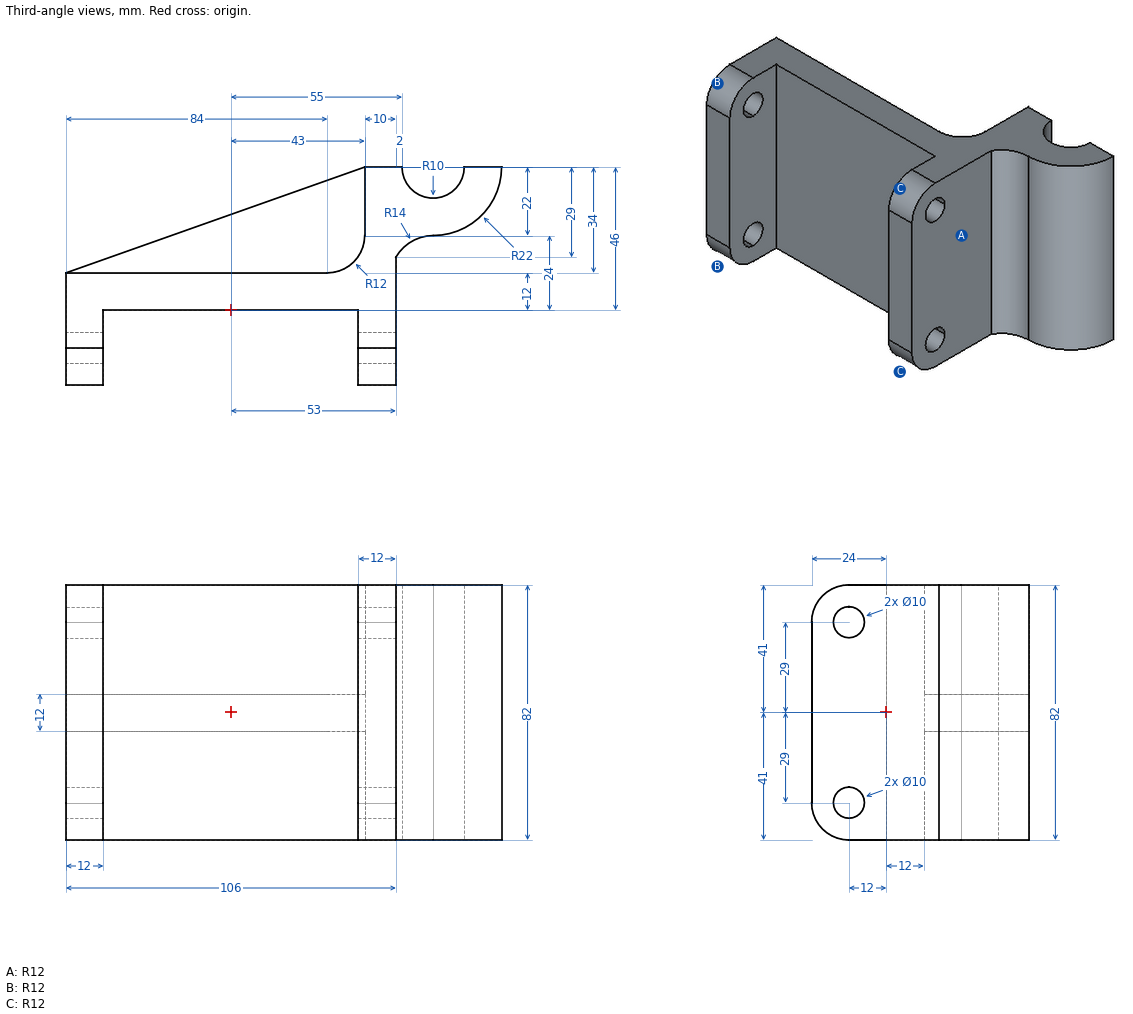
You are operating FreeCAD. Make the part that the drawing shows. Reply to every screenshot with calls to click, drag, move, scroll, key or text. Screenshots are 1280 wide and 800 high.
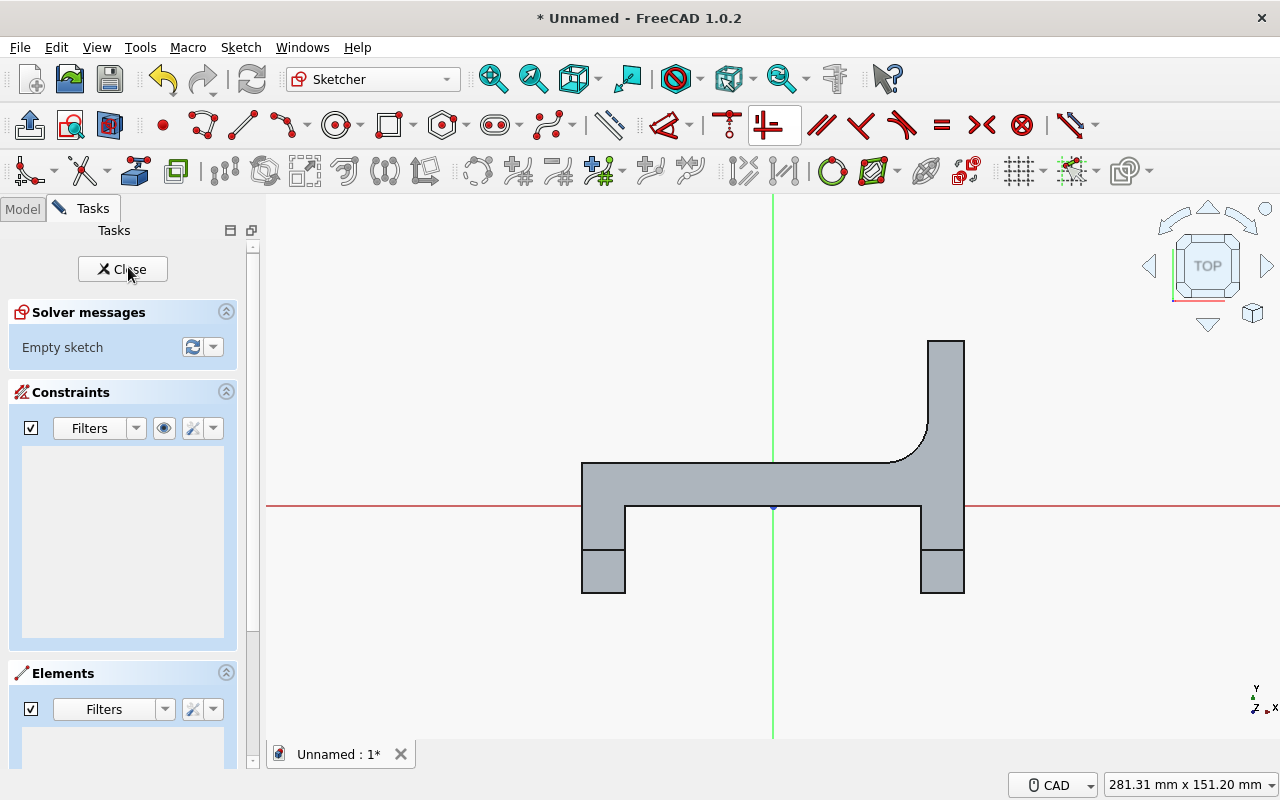
key(q)
key(s)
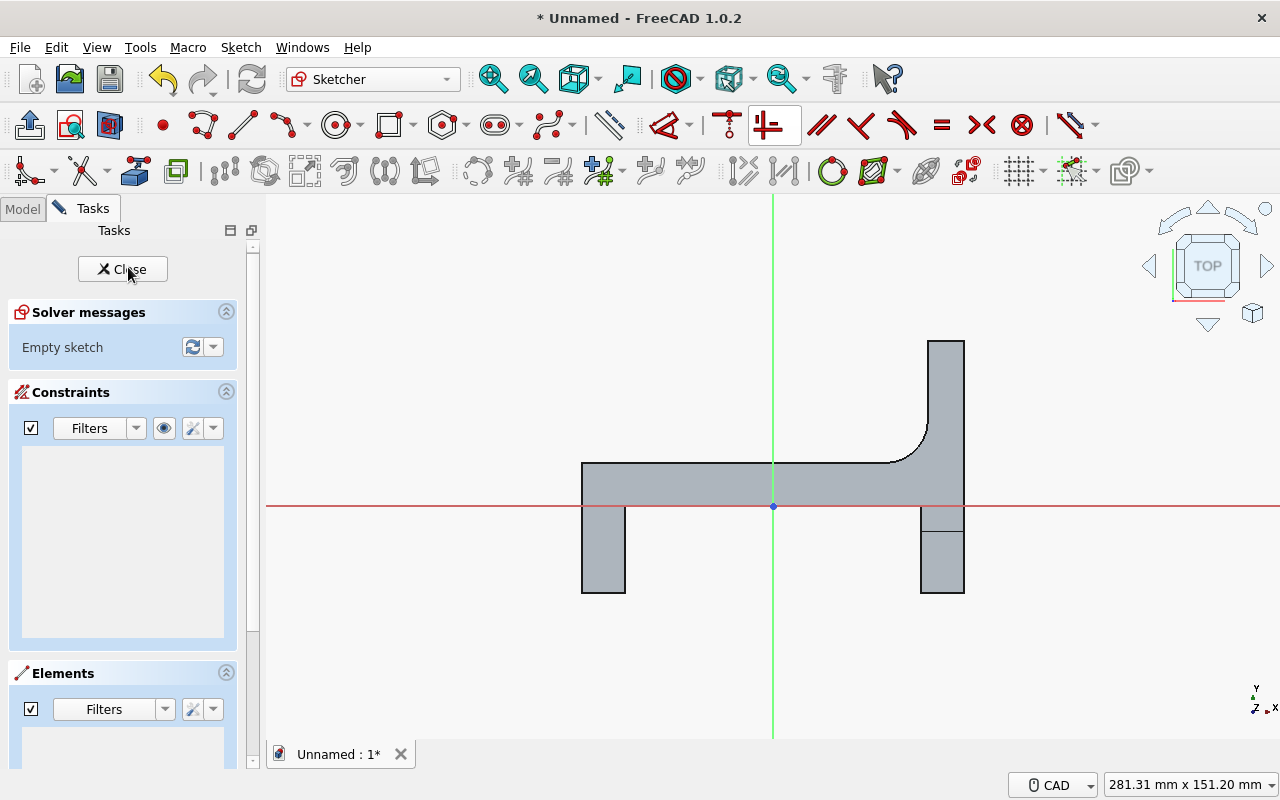
scroll(816, 371, up, 3)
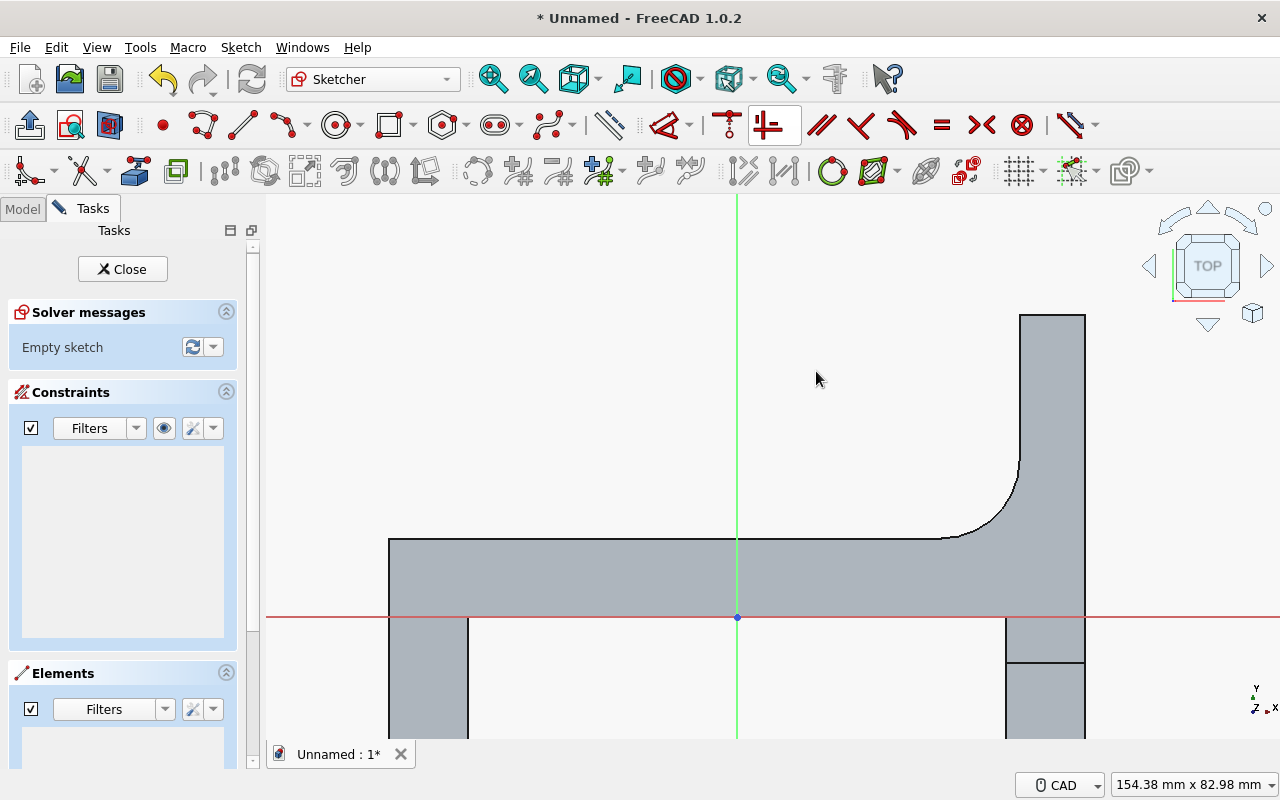
key(g)
key(m)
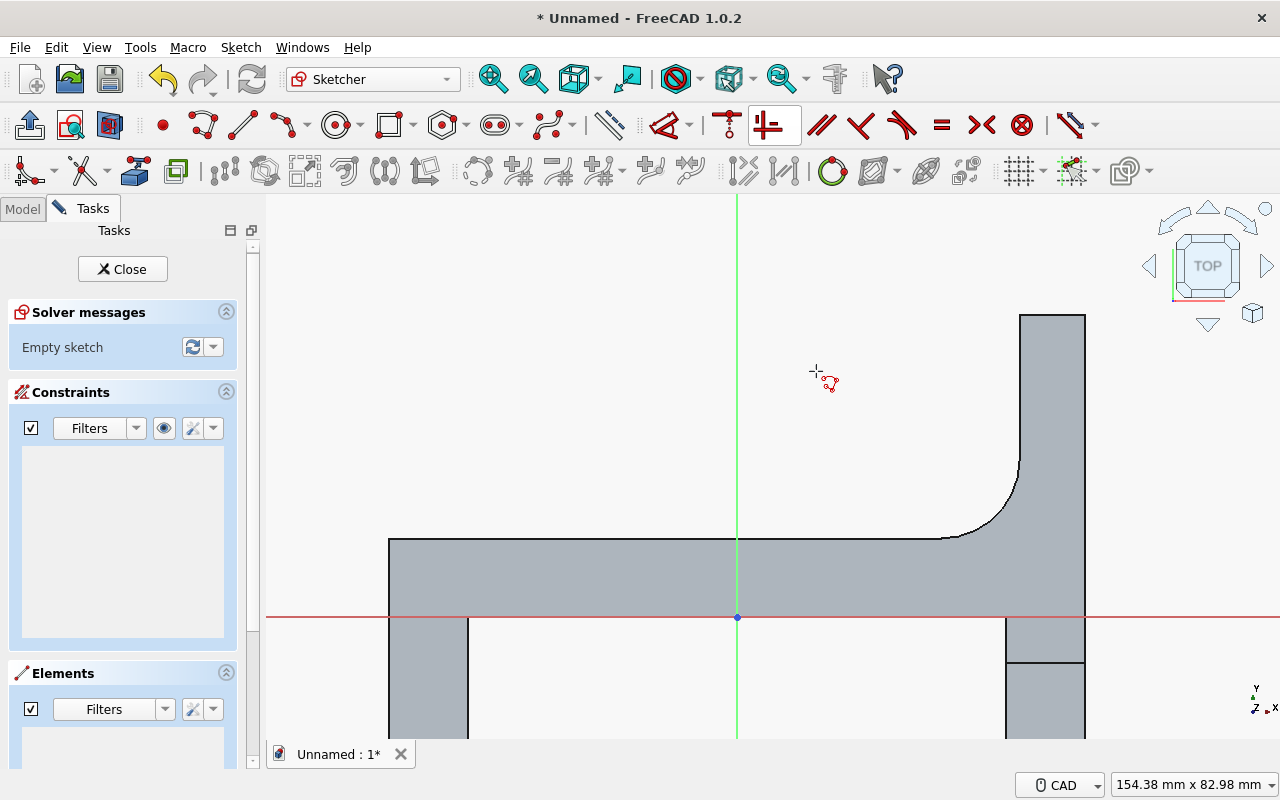
click(1020, 460)
click(1020, 315)
click(389, 539)
click(941, 539)
right_click(941, 539)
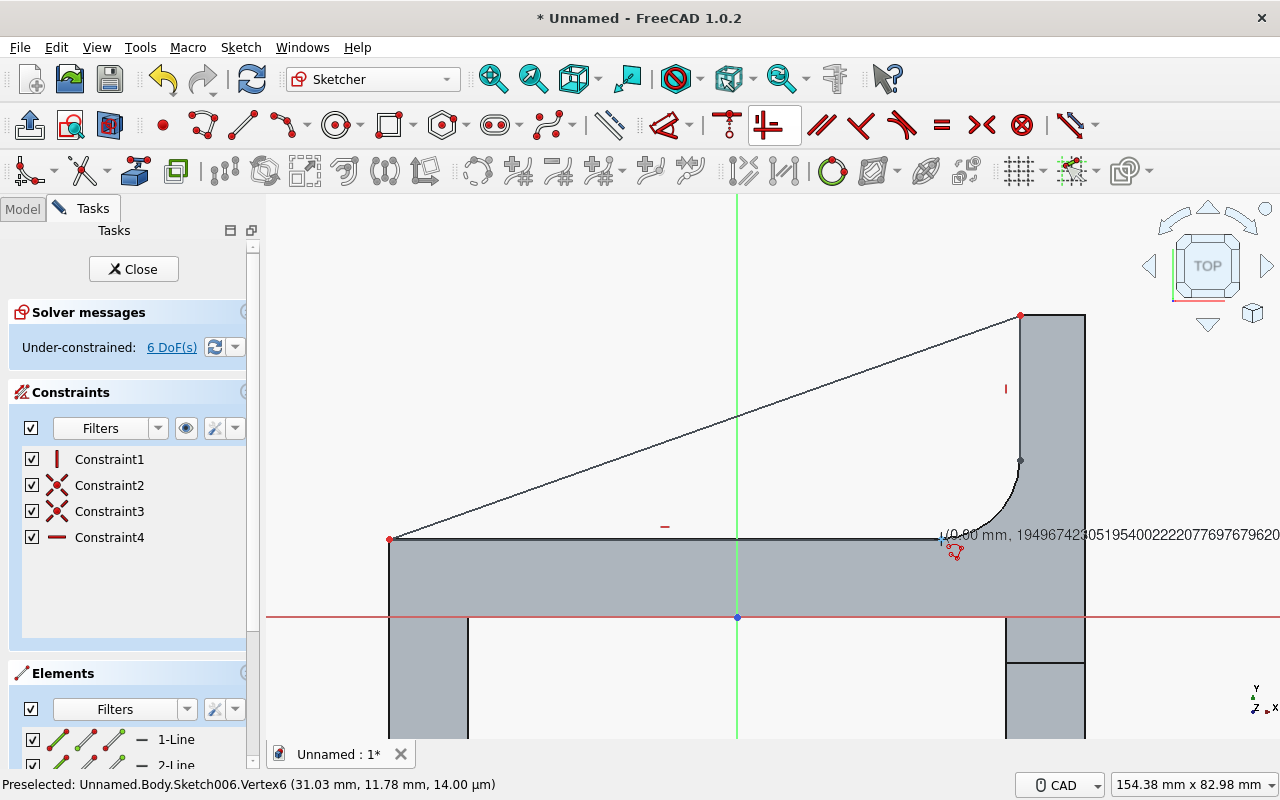
click(284, 126)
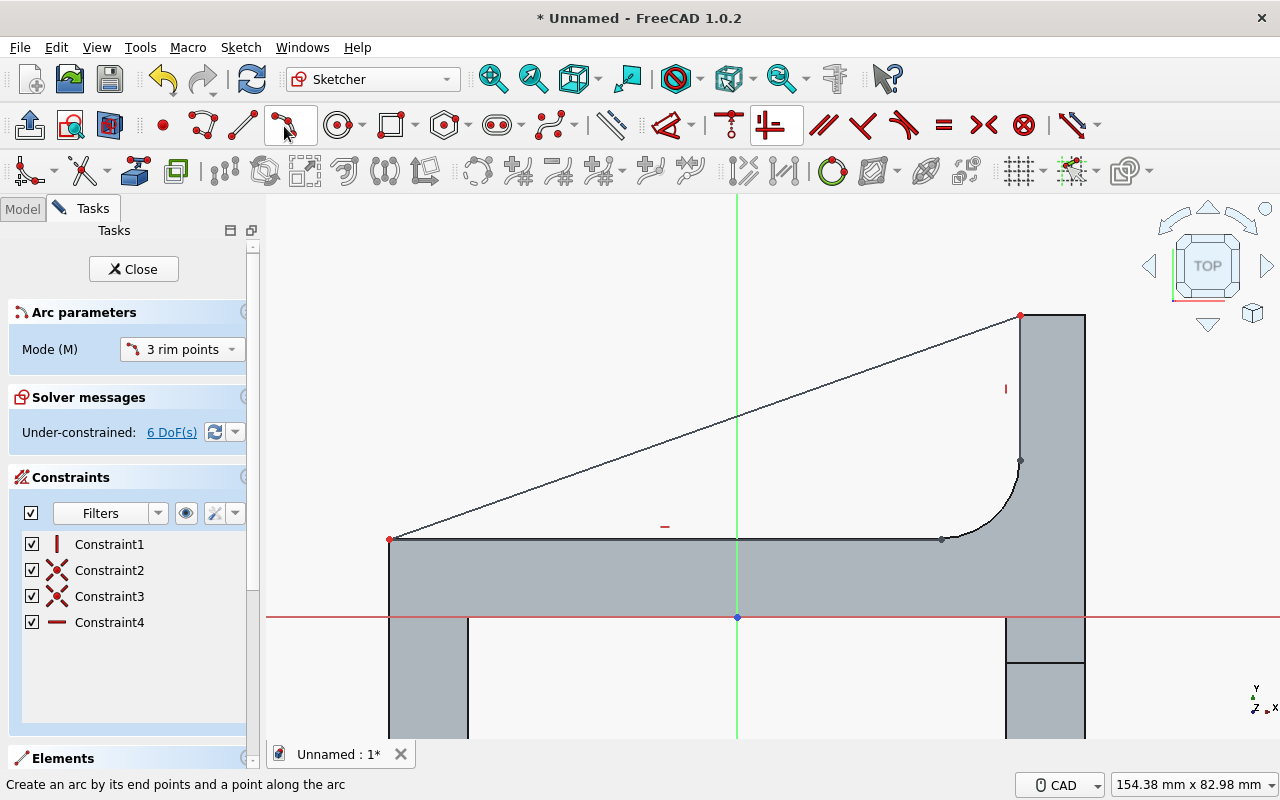
click(941, 540)
click(1020, 461)
click(997, 515)
key(Escape)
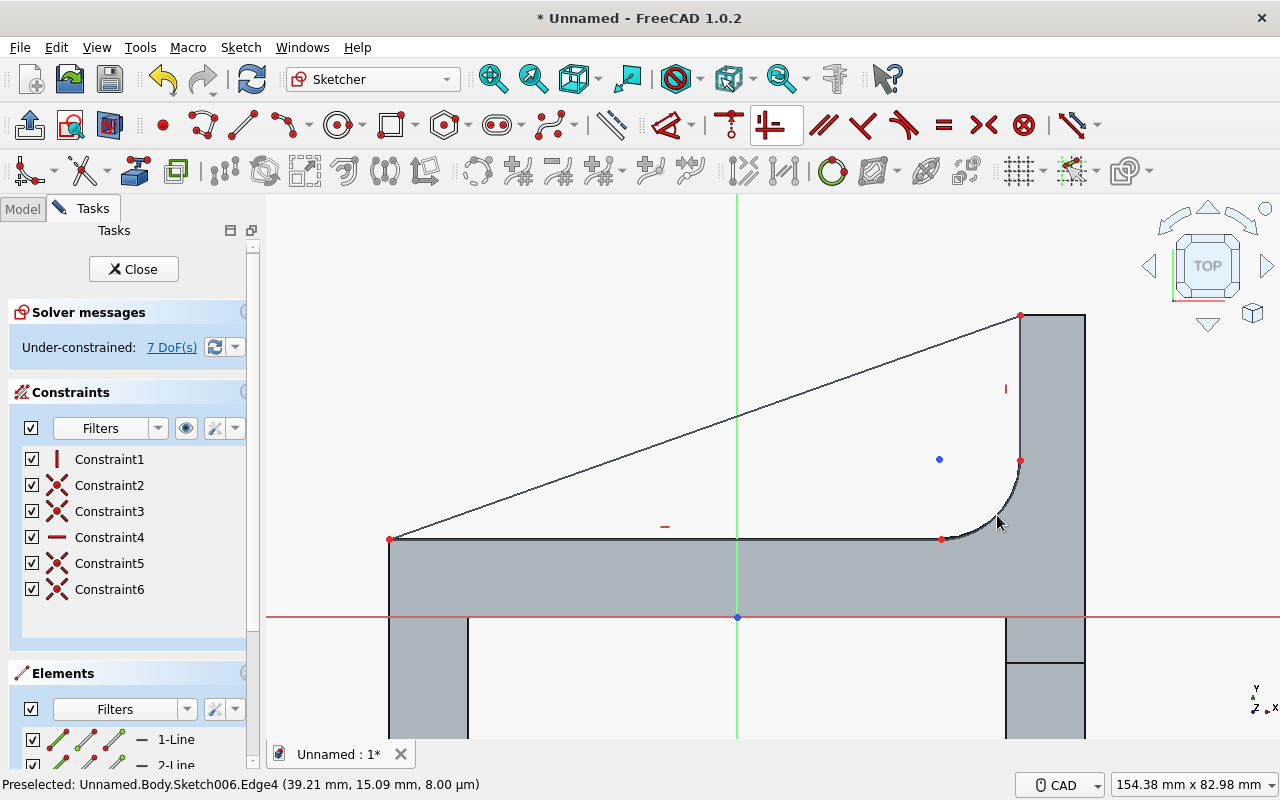
click(1020, 418)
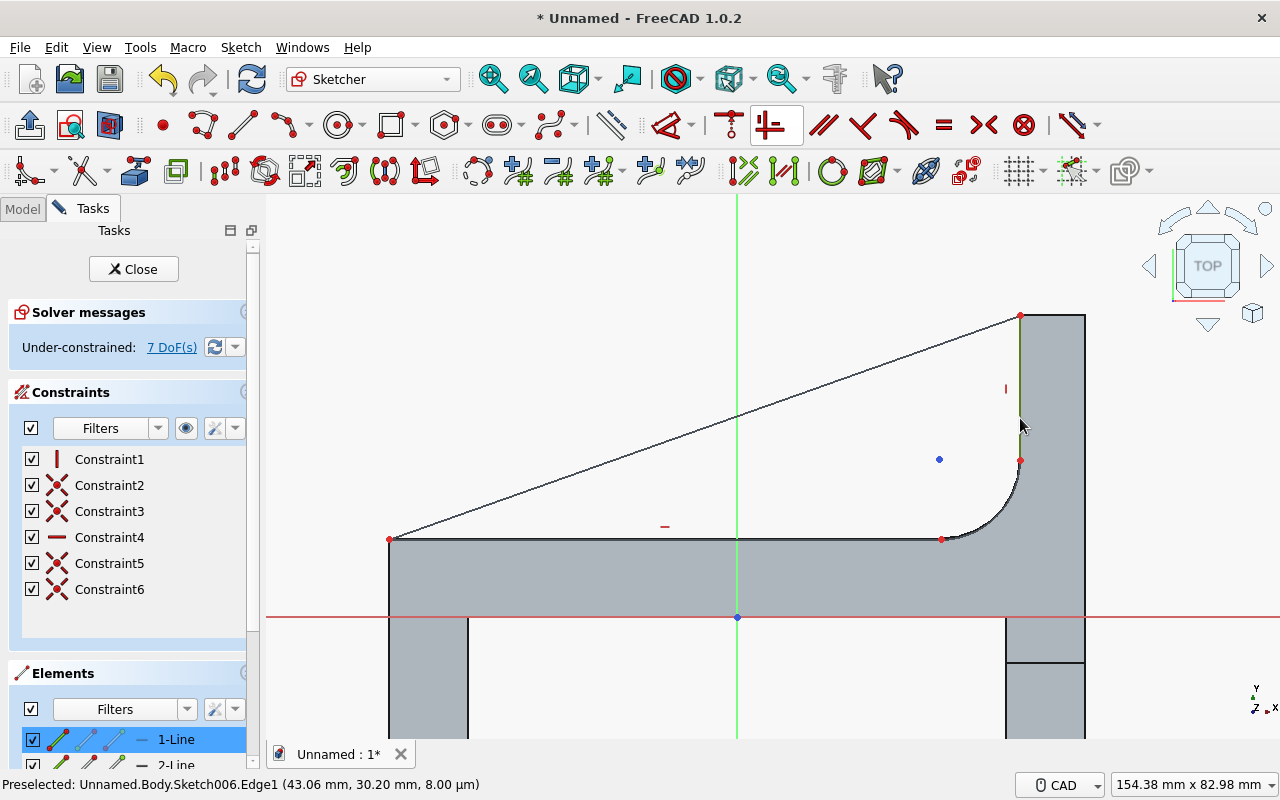
click(977, 531)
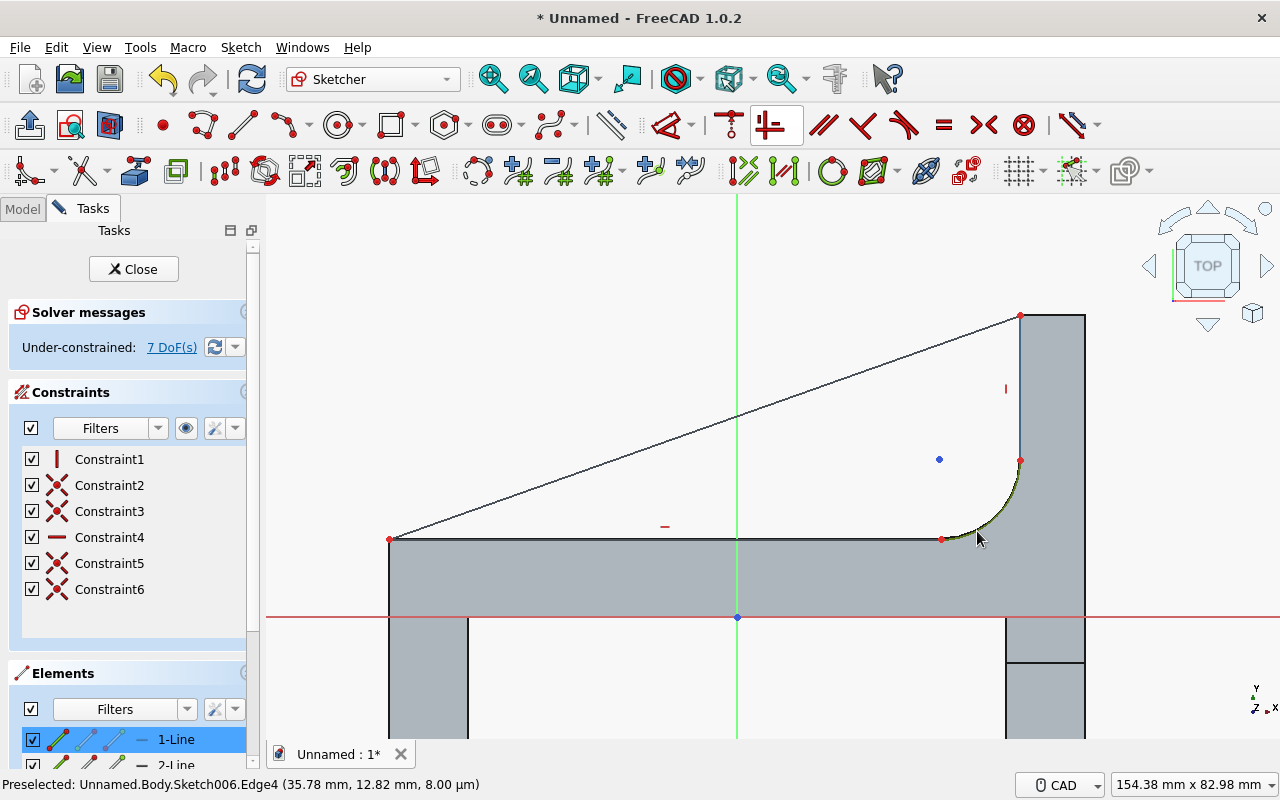
key(t)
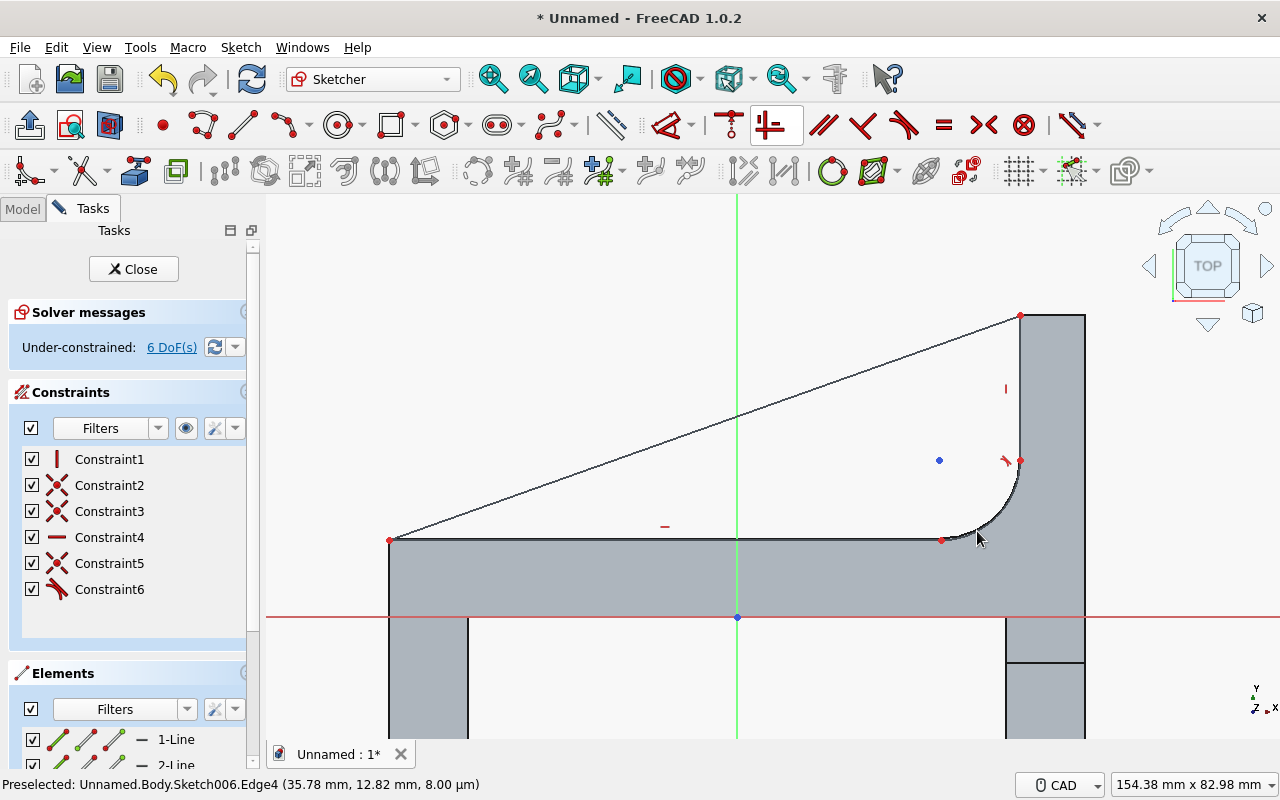
click(555, 540)